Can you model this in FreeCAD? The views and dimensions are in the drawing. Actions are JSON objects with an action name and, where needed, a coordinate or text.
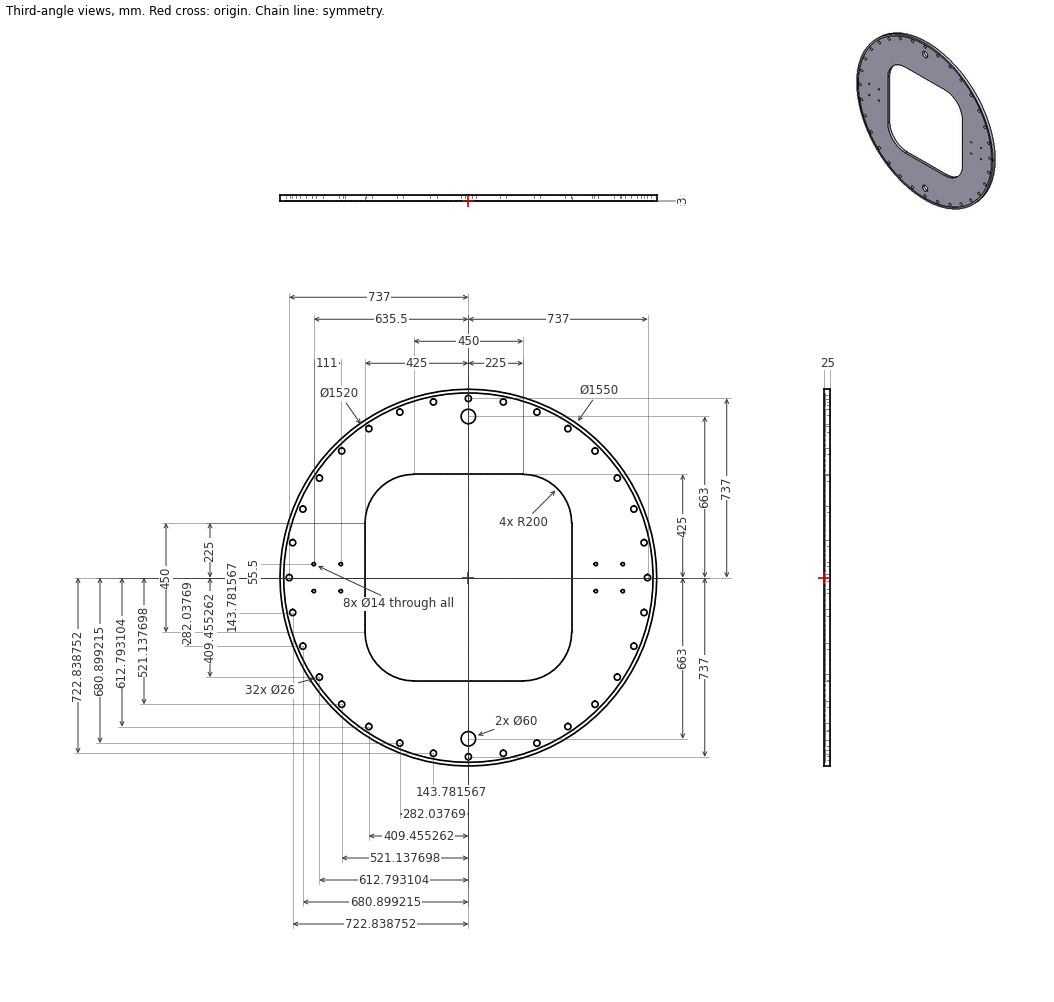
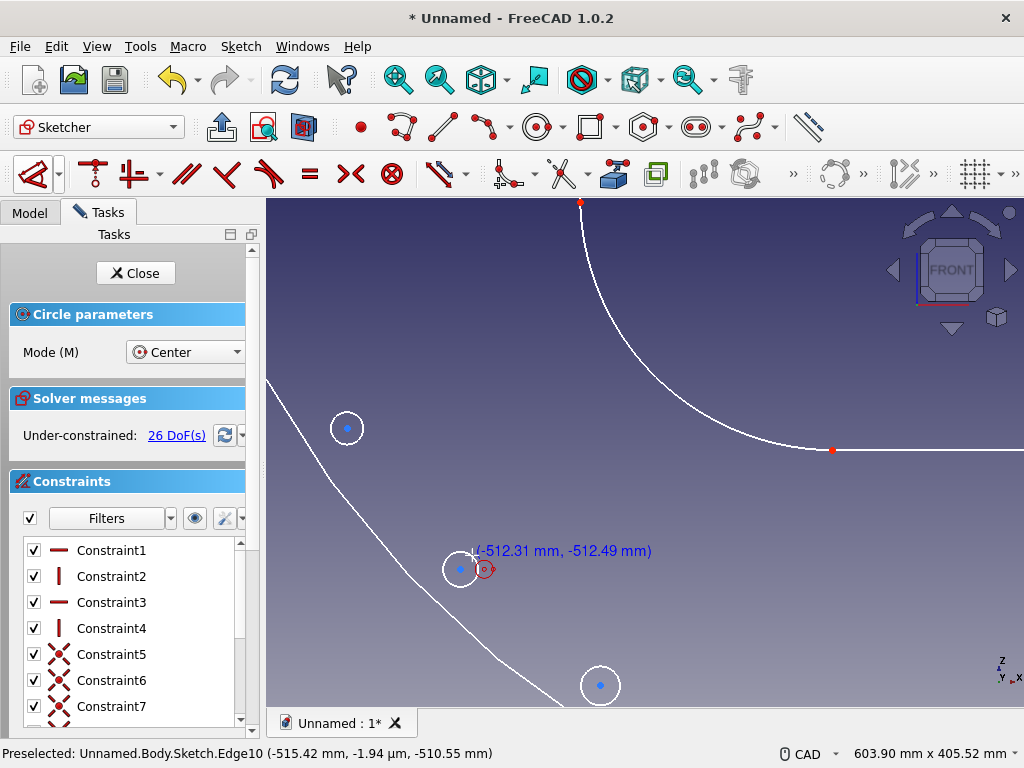
{"action": "scroll", "coordinate": [470, 559], "scroll_direction": "down", "scroll_amount": 9}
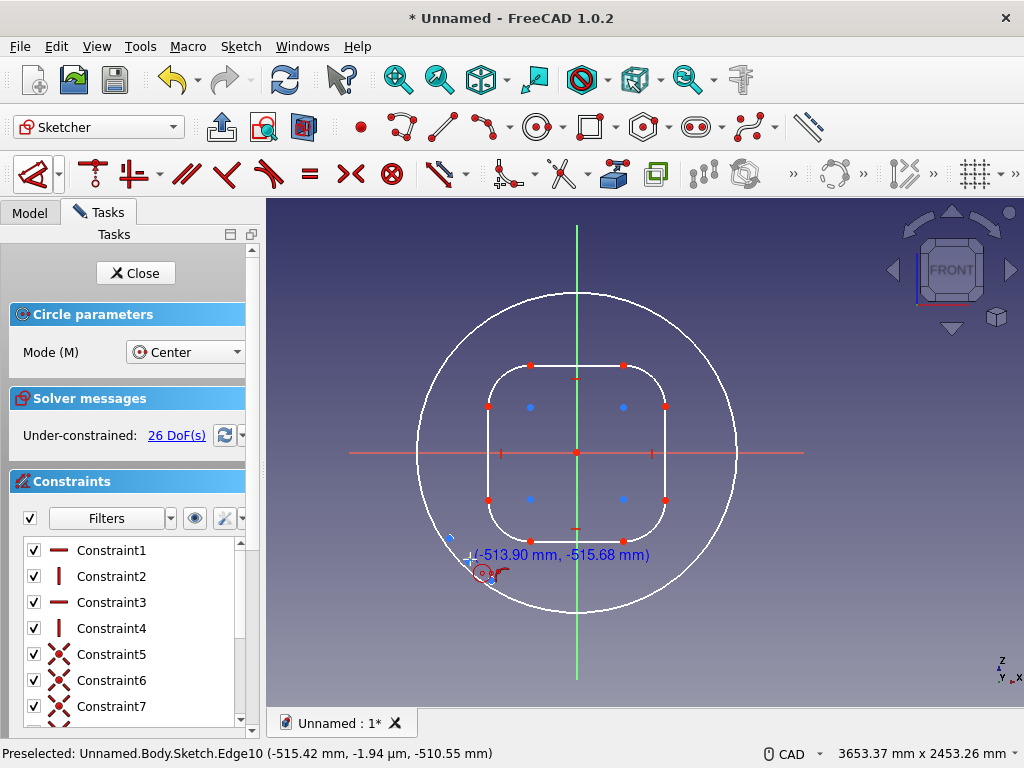
{"action": "scroll", "coordinate": [436, 511], "scroll_direction": "up", "scroll_amount": 11}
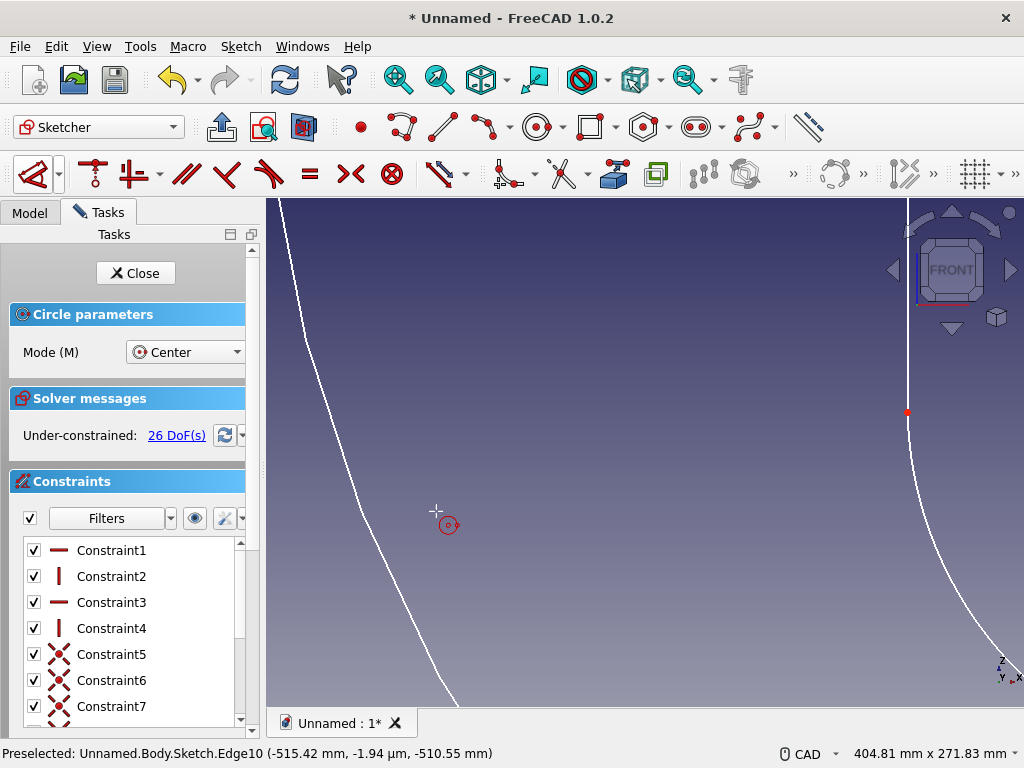
{"action": "scroll", "coordinate": [436, 511], "scroll_direction": "down", "scroll_amount": 11}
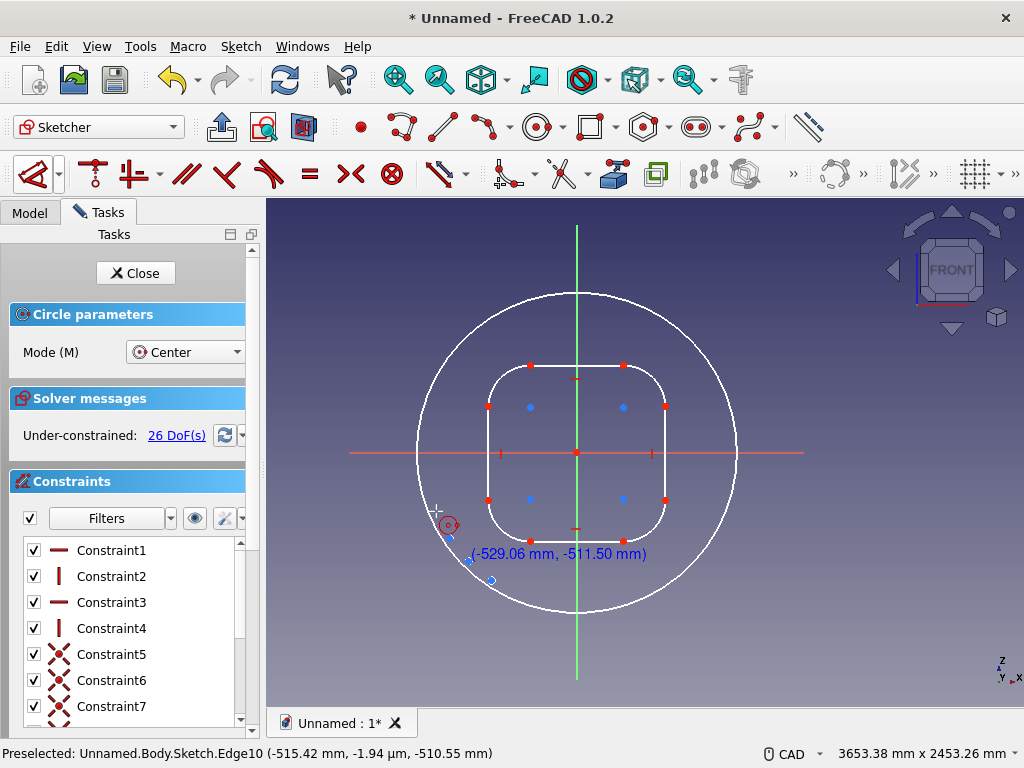
{"action": "scroll", "coordinate": [436, 511], "scroll_direction": "up", "scroll_amount": 4}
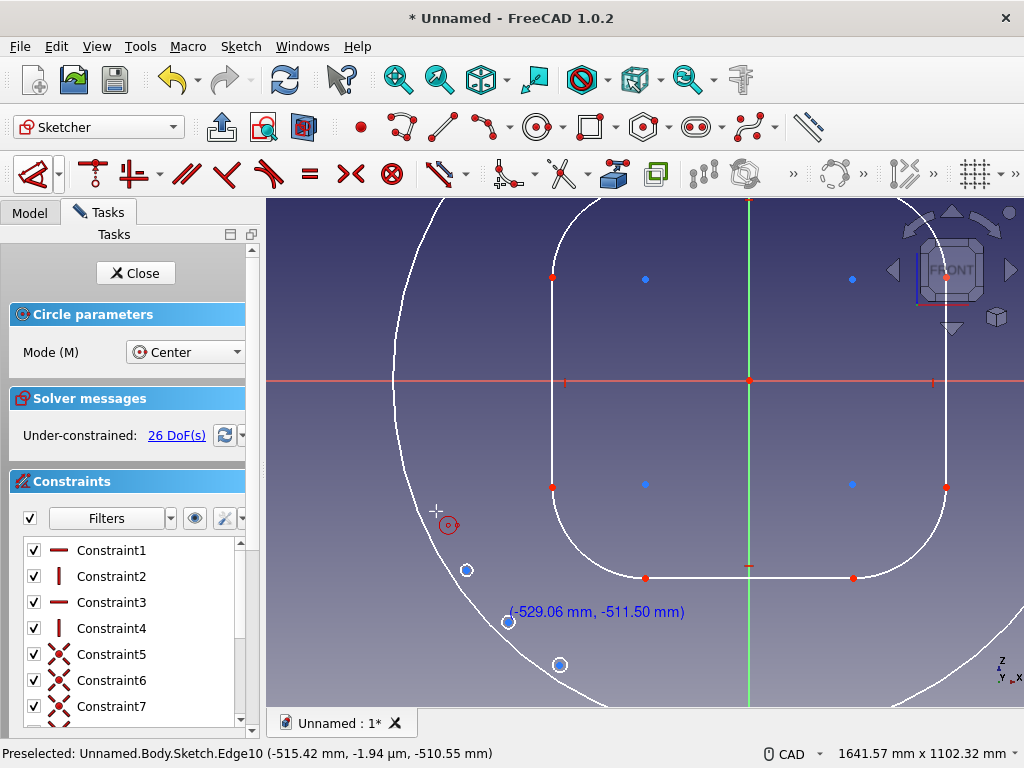
{"action": "left_click", "coordinate": [435, 511]}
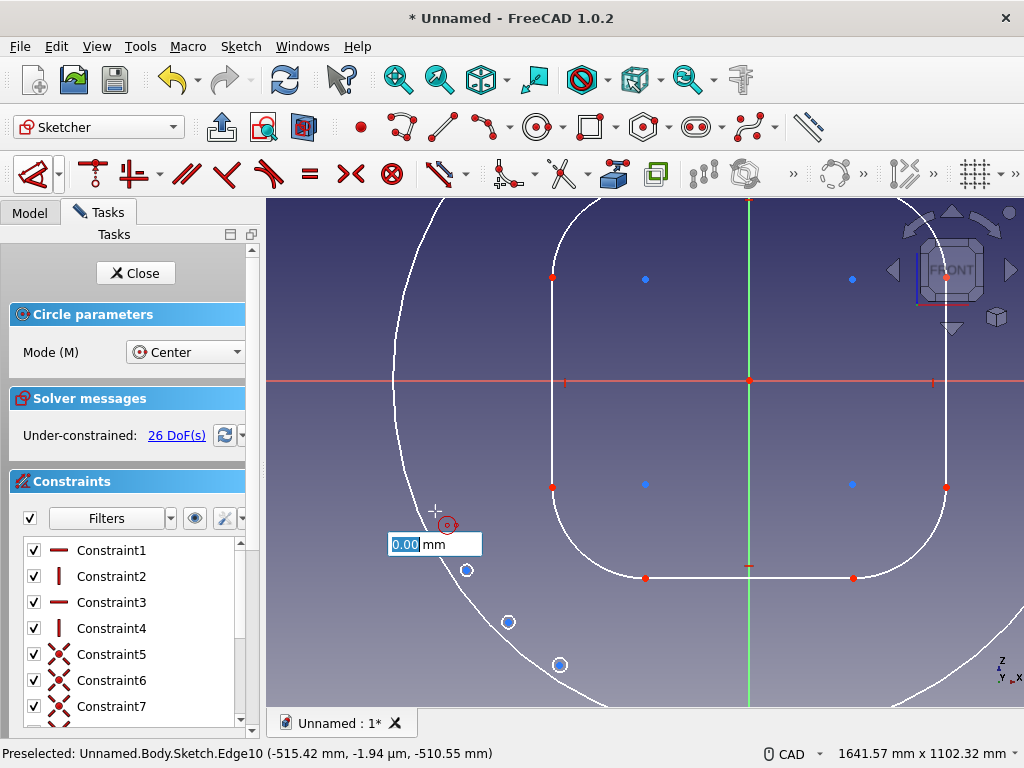
{"action": "scroll", "coordinate": [439, 507], "scroll_direction": "up", "scroll_amount": 5}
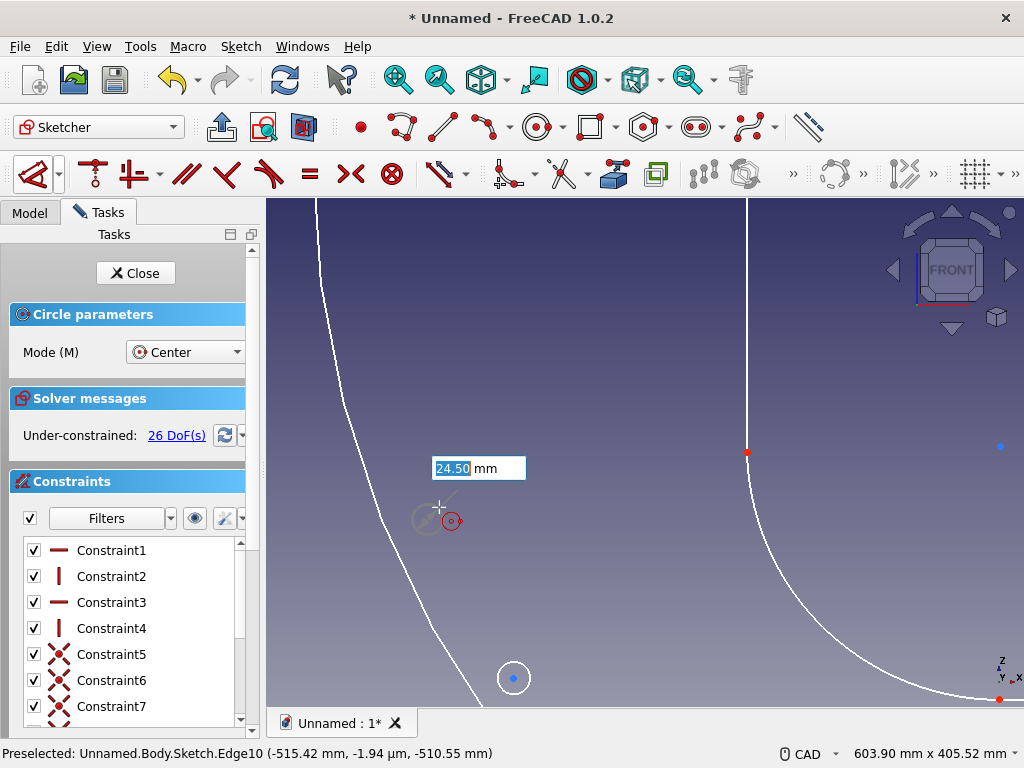
{"action": "left_click", "coordinate": [439, 505]}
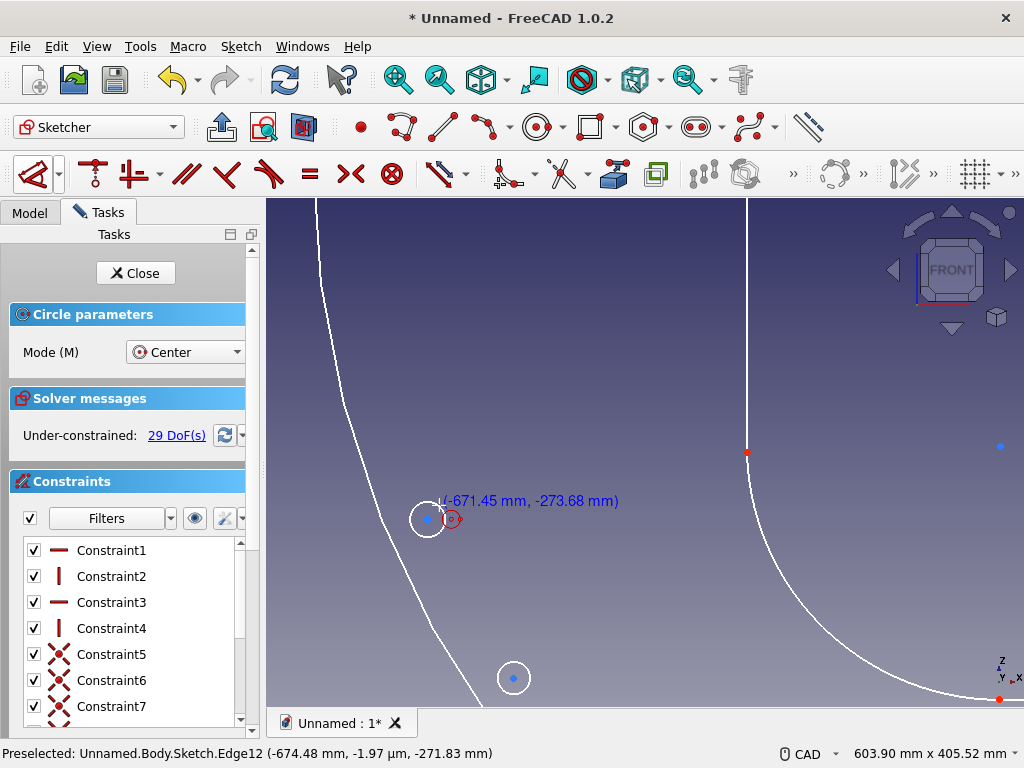
{"action": "scroll", "coordinate": [375, 343], "scroll_direction": "up", "scroll_amount": 2}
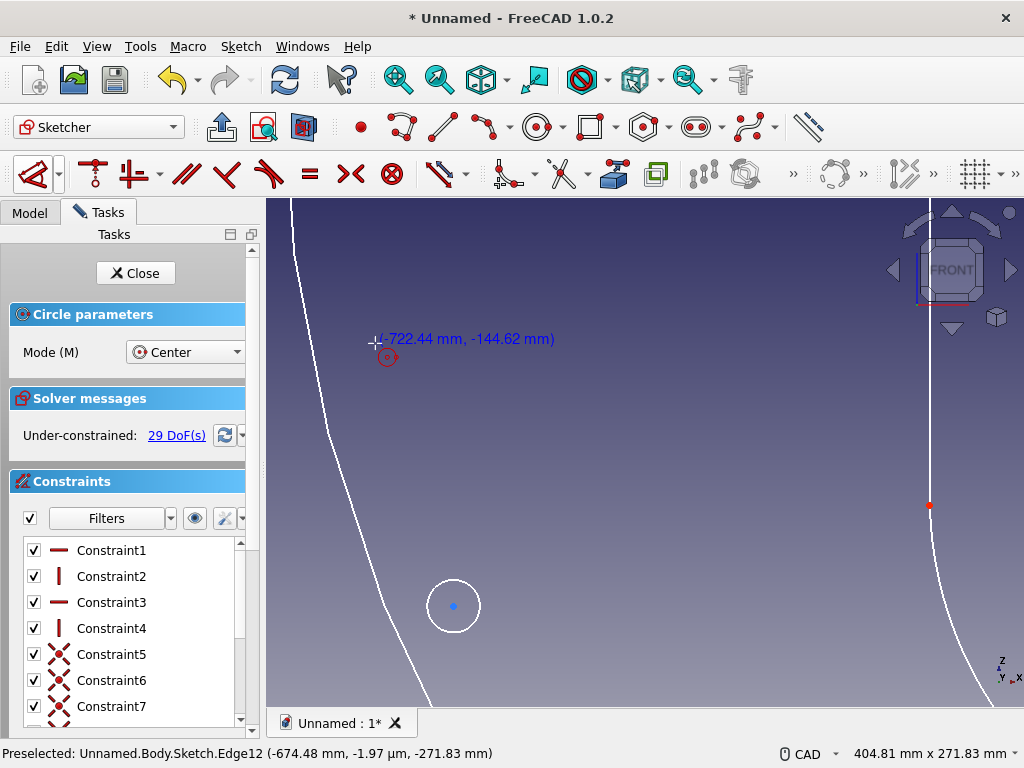
{"action": "scroll", "coordinate": [433, 500], "scroll_direction": "down", "scroll_amount": 11}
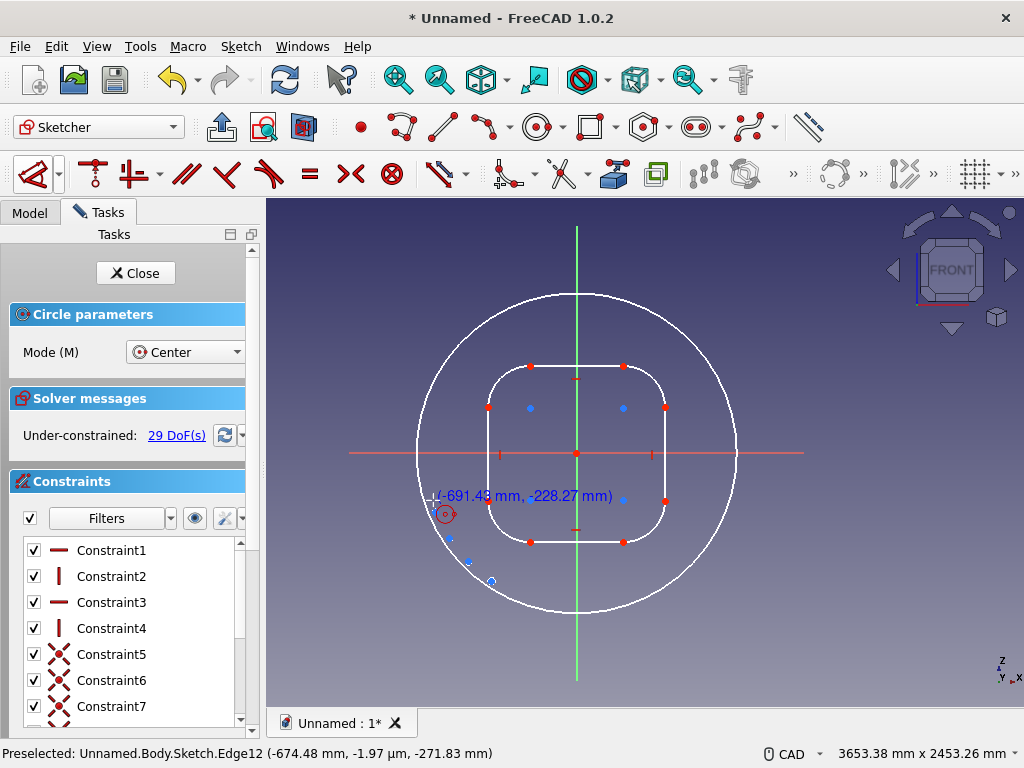
{"action": "scroll", "coordinate": [427, 483], "scroll_direction": "up", "scroll_amount": 4}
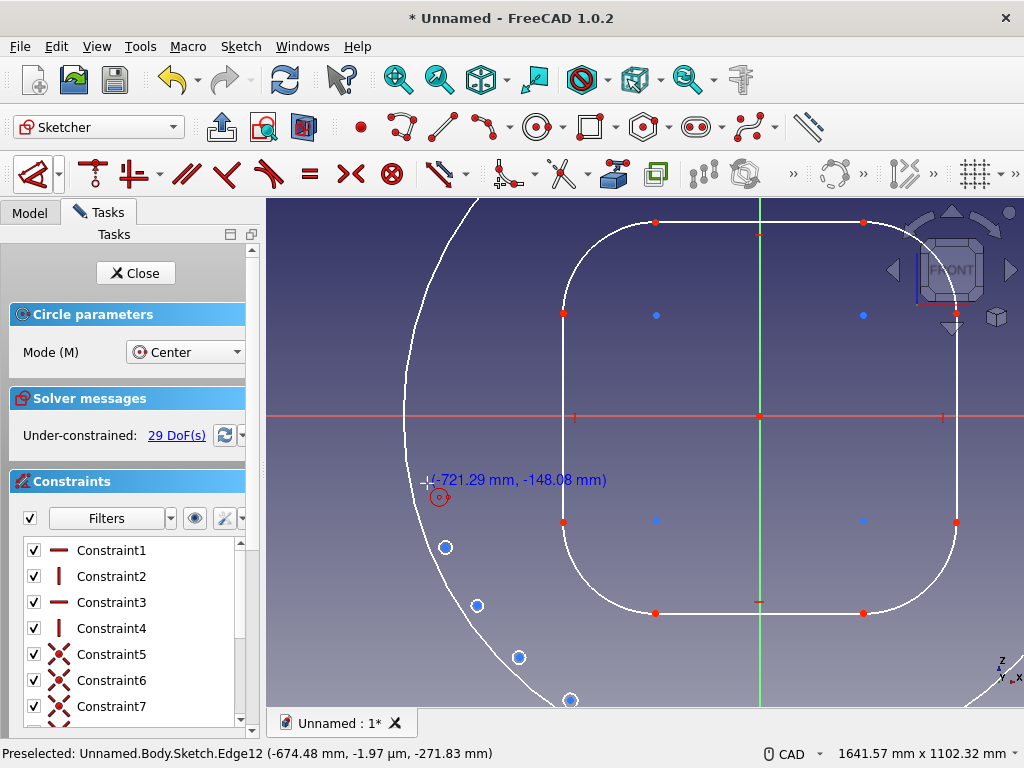
{"action": "left_click", "coordinate": [426, 483]}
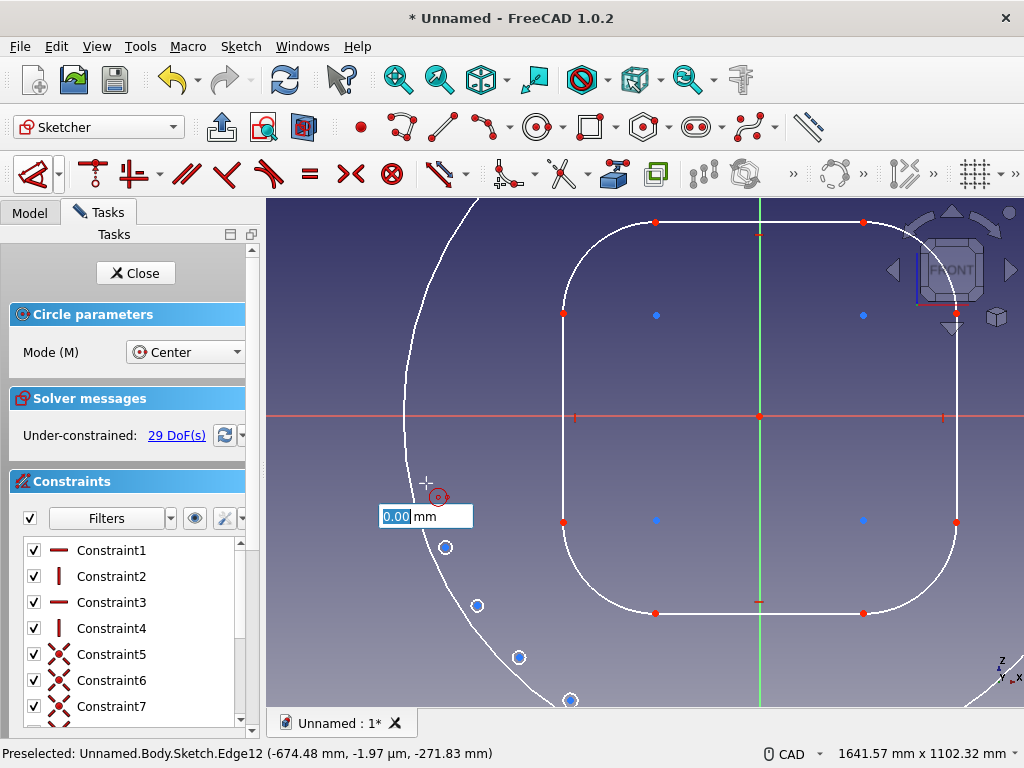
{"action": "scroll", "coordinate": [430, 478], "scroll_direction": "up", "scroll_amount": 5}